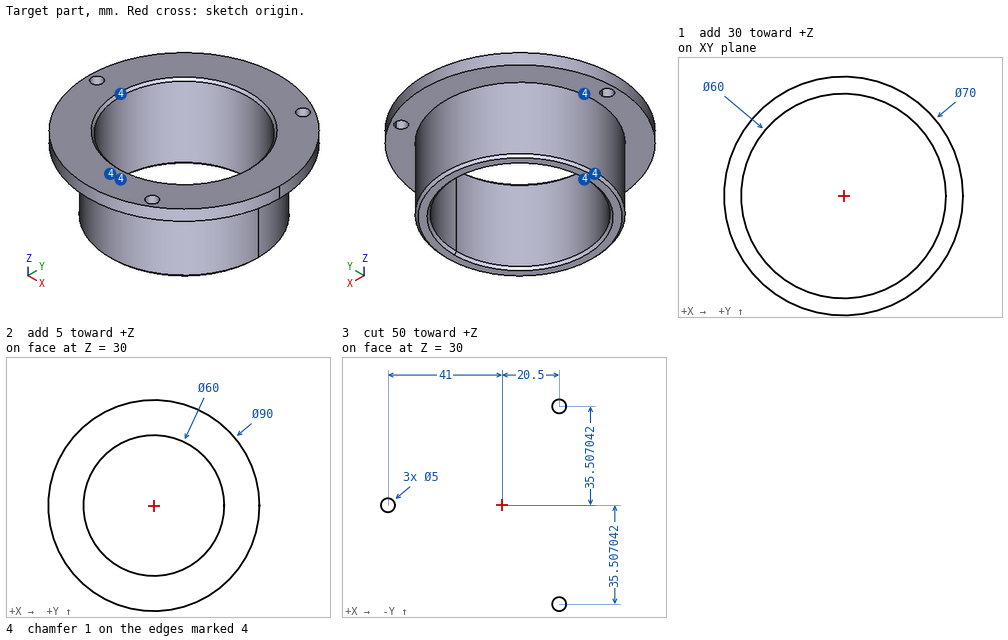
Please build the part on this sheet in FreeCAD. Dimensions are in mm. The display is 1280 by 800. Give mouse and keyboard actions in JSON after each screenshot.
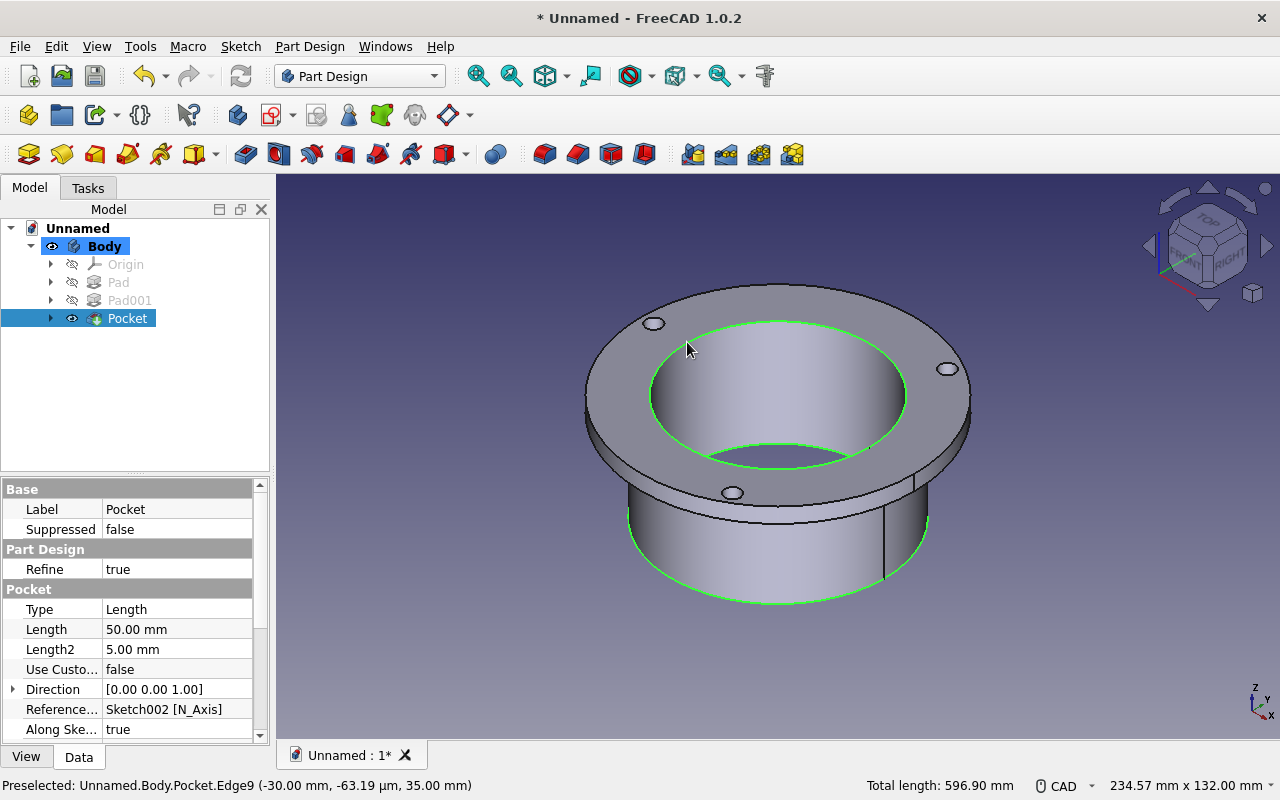
{"action": "left_click", "coordinate": [578, 154]}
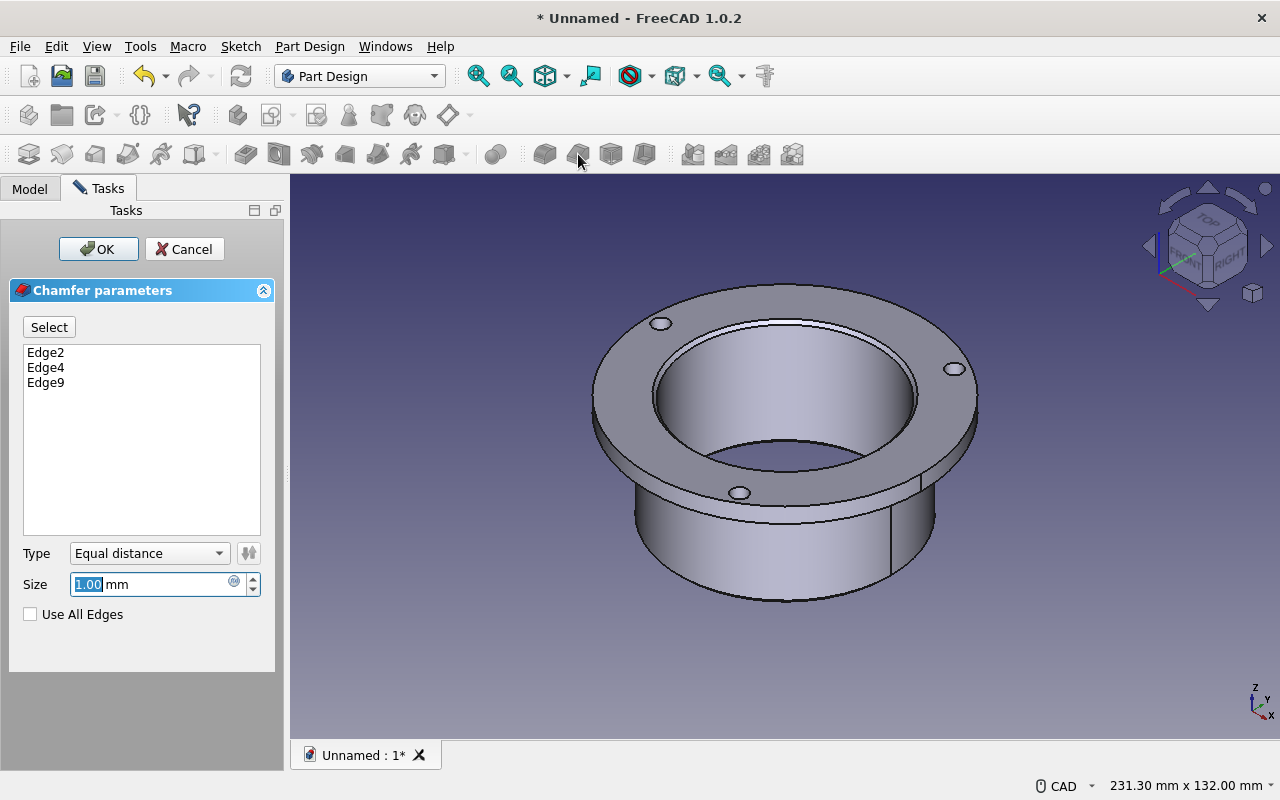
{"action": "type", "text": "1"}
{"action": "key", "text": "Tab"}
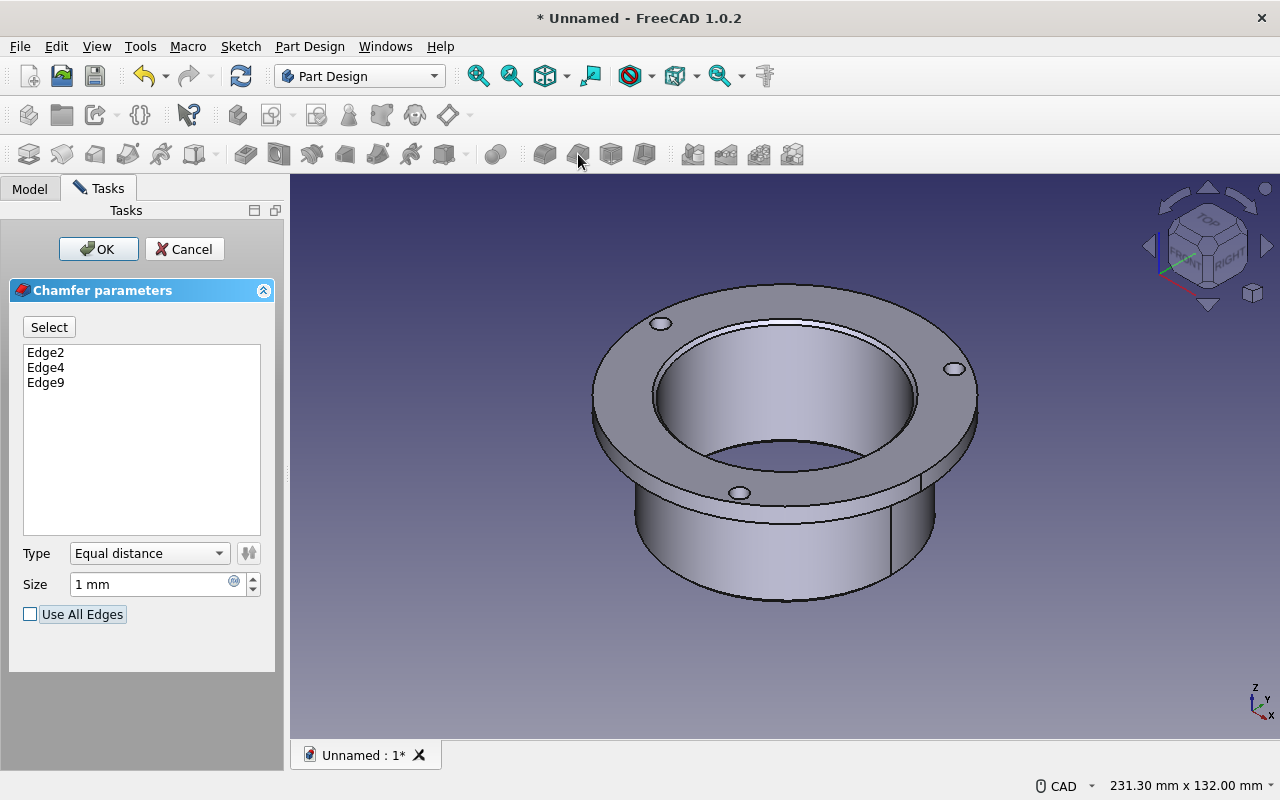
{"action": "left_click", "coordinate": [99, 249]}